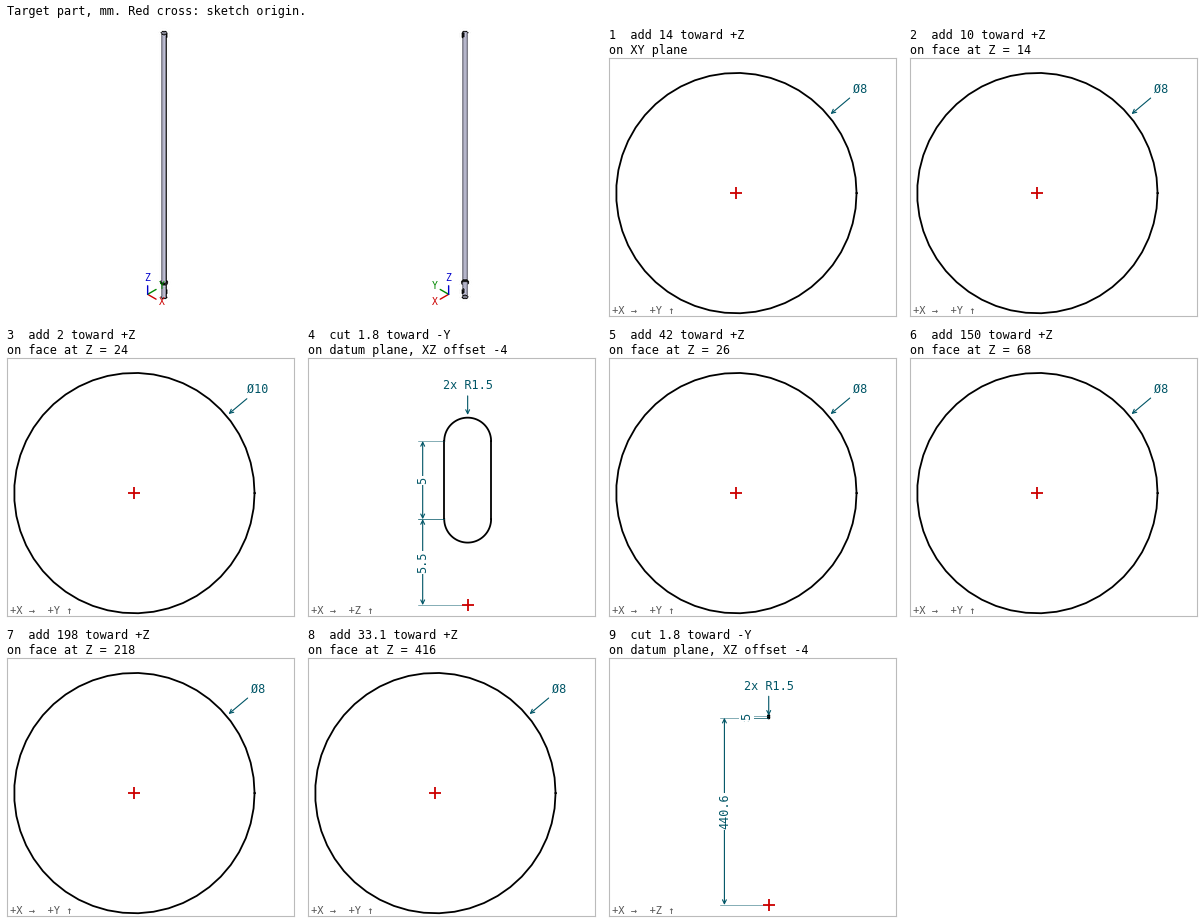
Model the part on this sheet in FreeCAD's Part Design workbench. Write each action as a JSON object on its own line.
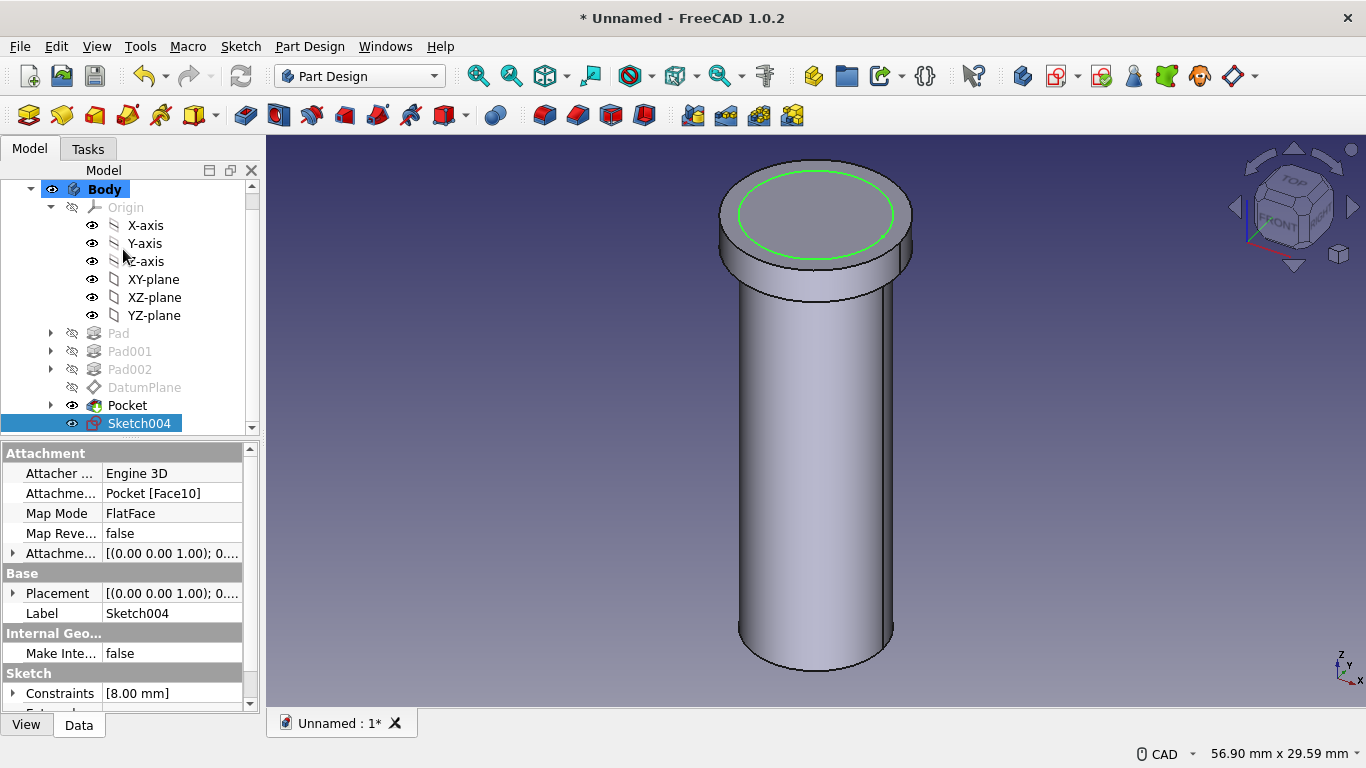
{"action": "left_click", "coordinate": [29, 116]}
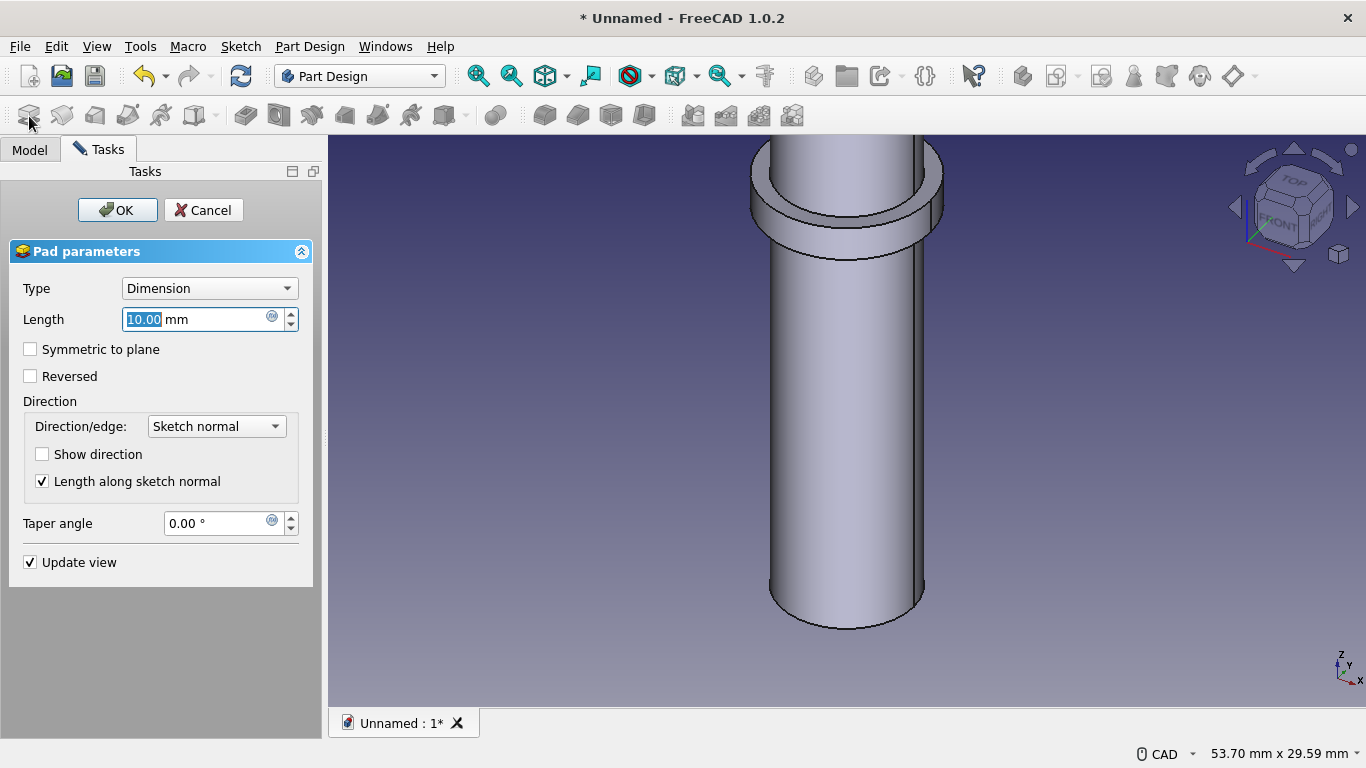
{"action": "type", "text": "42"}
{"action": "key", "text": "Tab"}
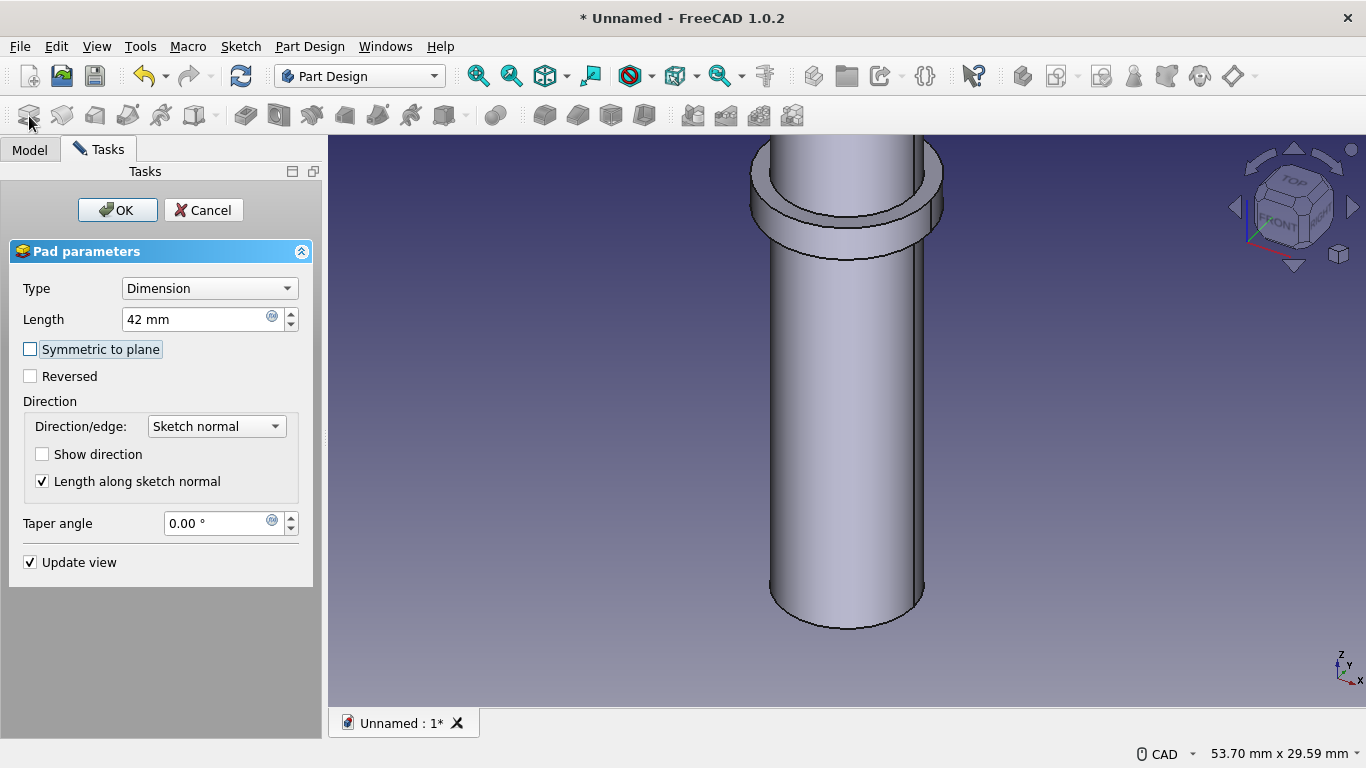
{"action": "left_click", "coordinate": [118, 210]}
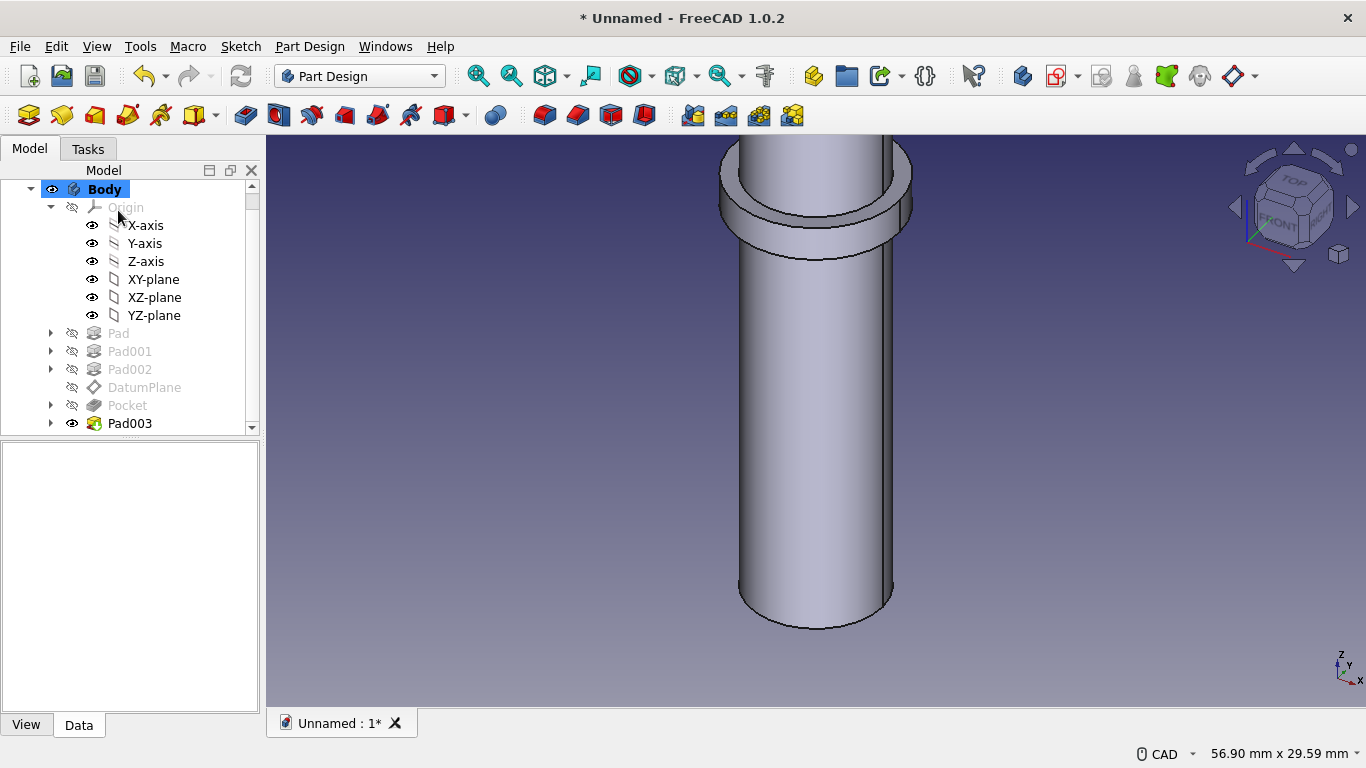
{"action": "left_click", "coordinate": [479, 76]}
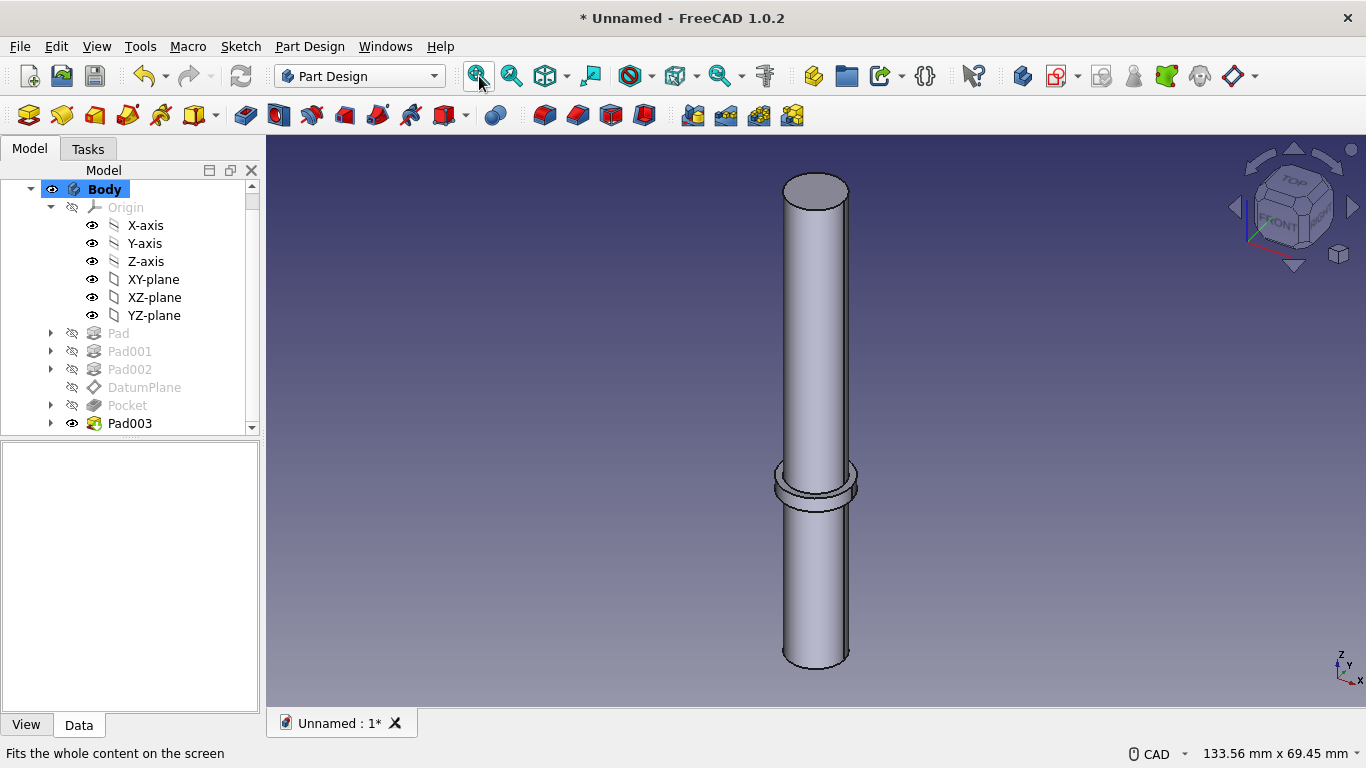
{"action": "left_click", "coordinate": [816, 191]}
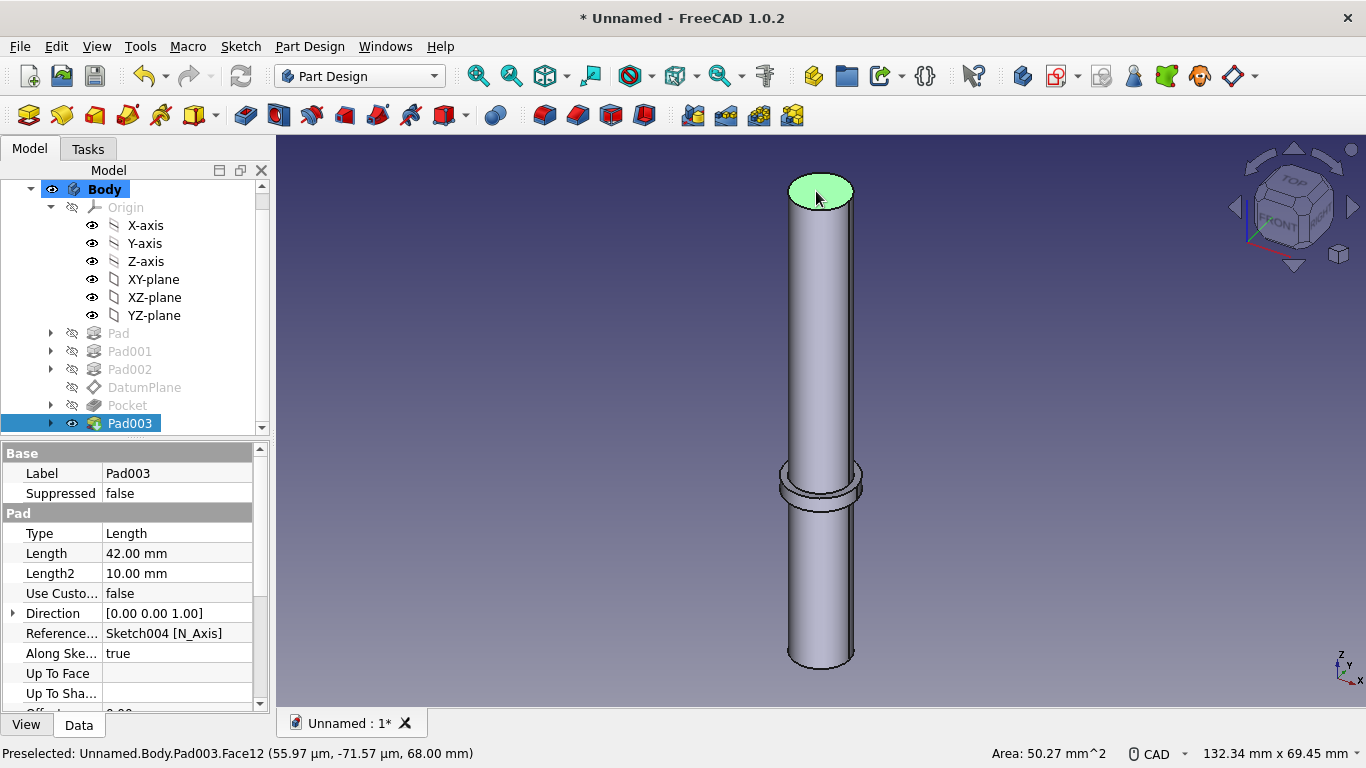
{"action": "left_click", "coordinate": [1056, 76]}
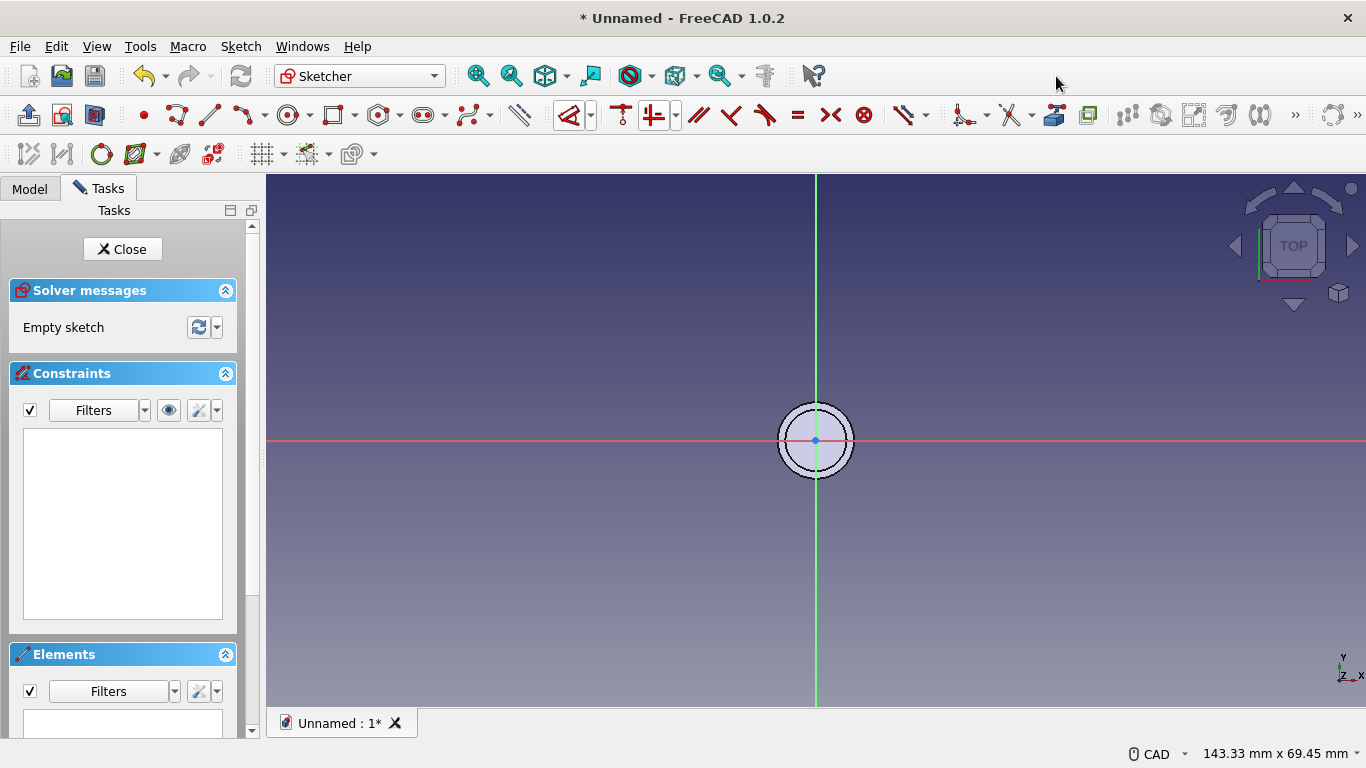
{"action": "scroll", "coordinate": [829, 440], "scroll_direction": "up", "scroll_amount": 9}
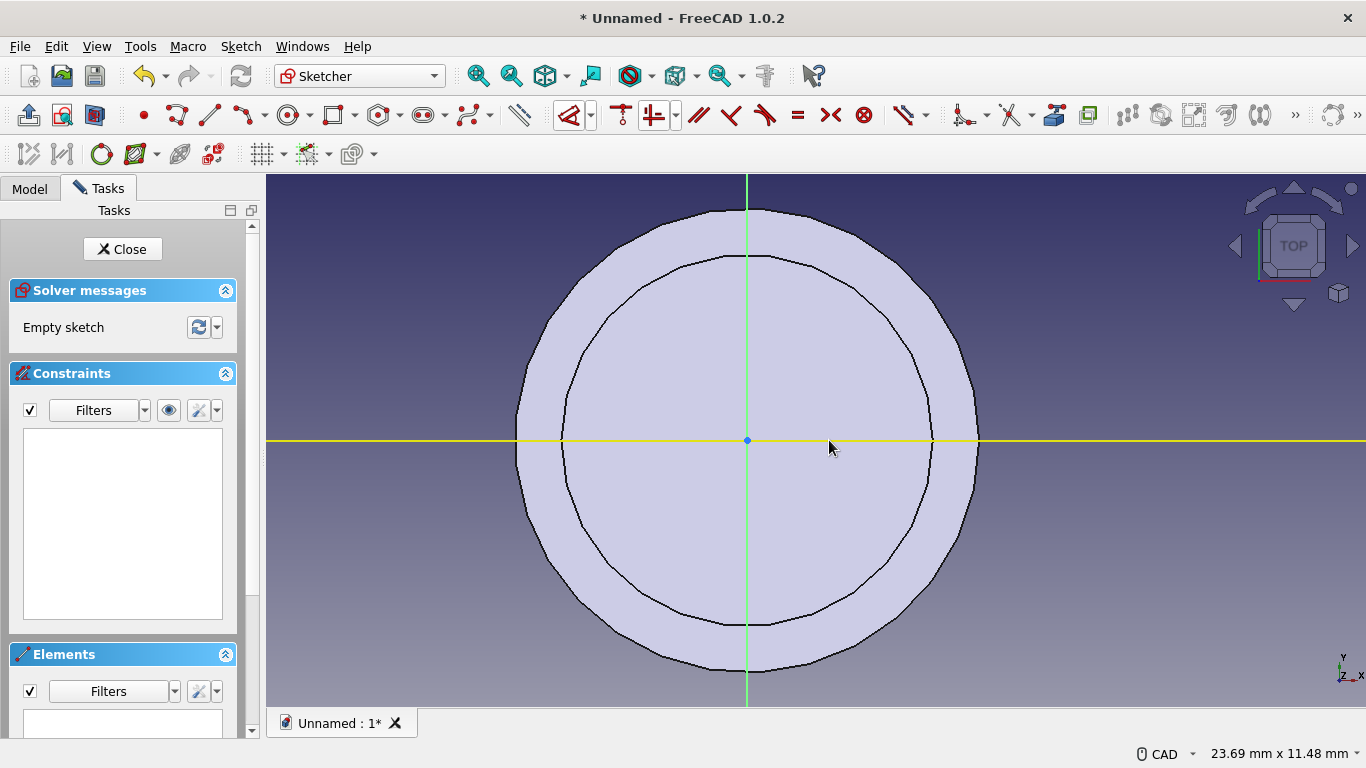
{"action": "left_click", "coordinate": [288, 116]}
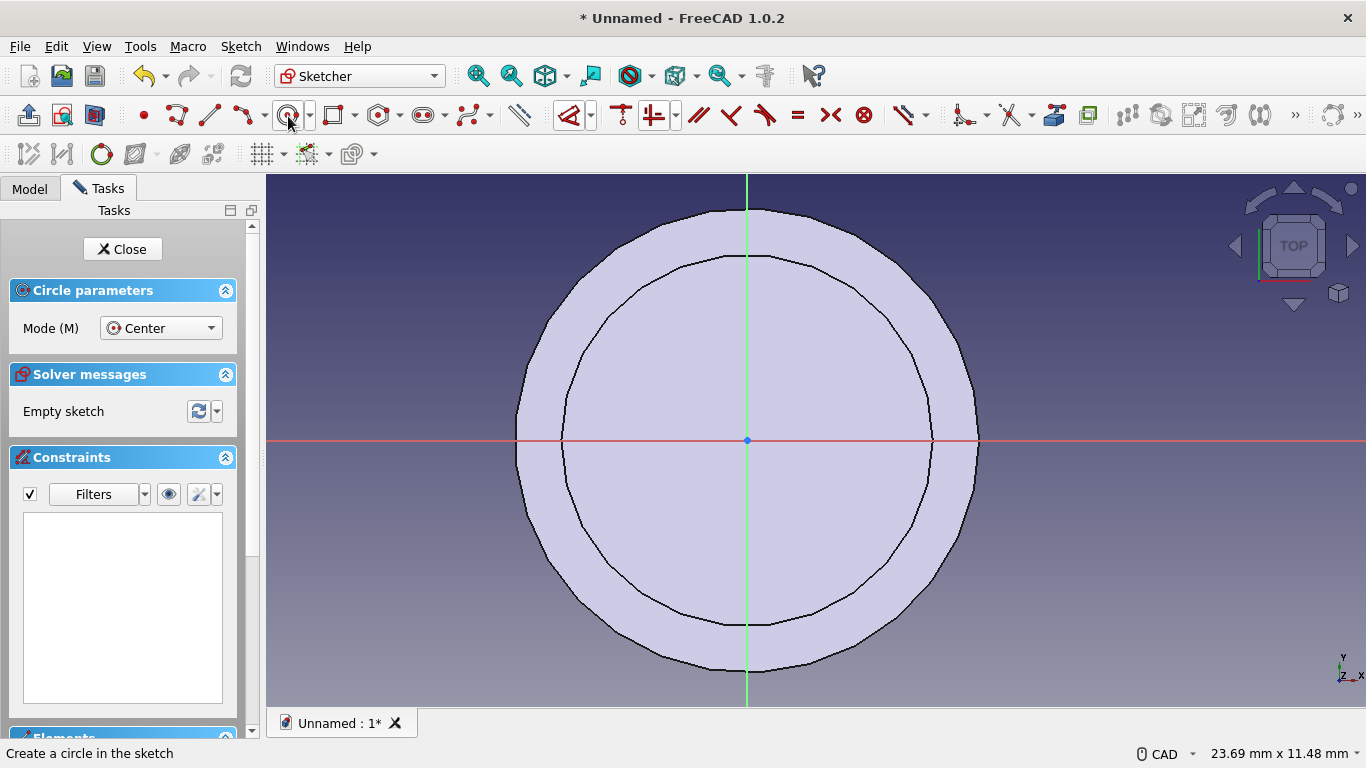
{"action": "left_click", "coordinate": [747, 440]}
{"action": "left_click", "coordinate": [878, 309]}
{"action": "key", "text": "Escape"}